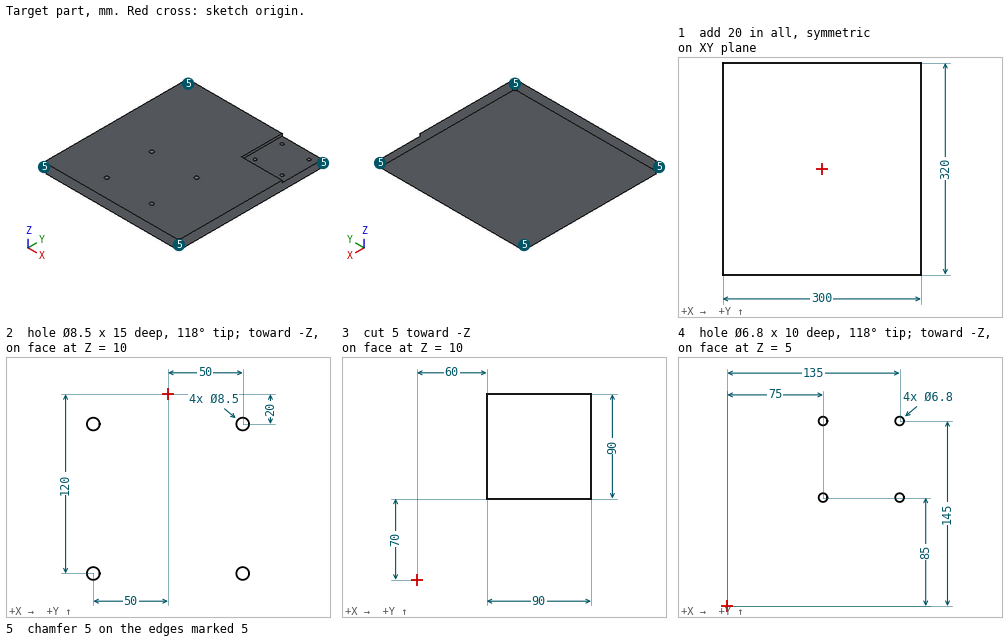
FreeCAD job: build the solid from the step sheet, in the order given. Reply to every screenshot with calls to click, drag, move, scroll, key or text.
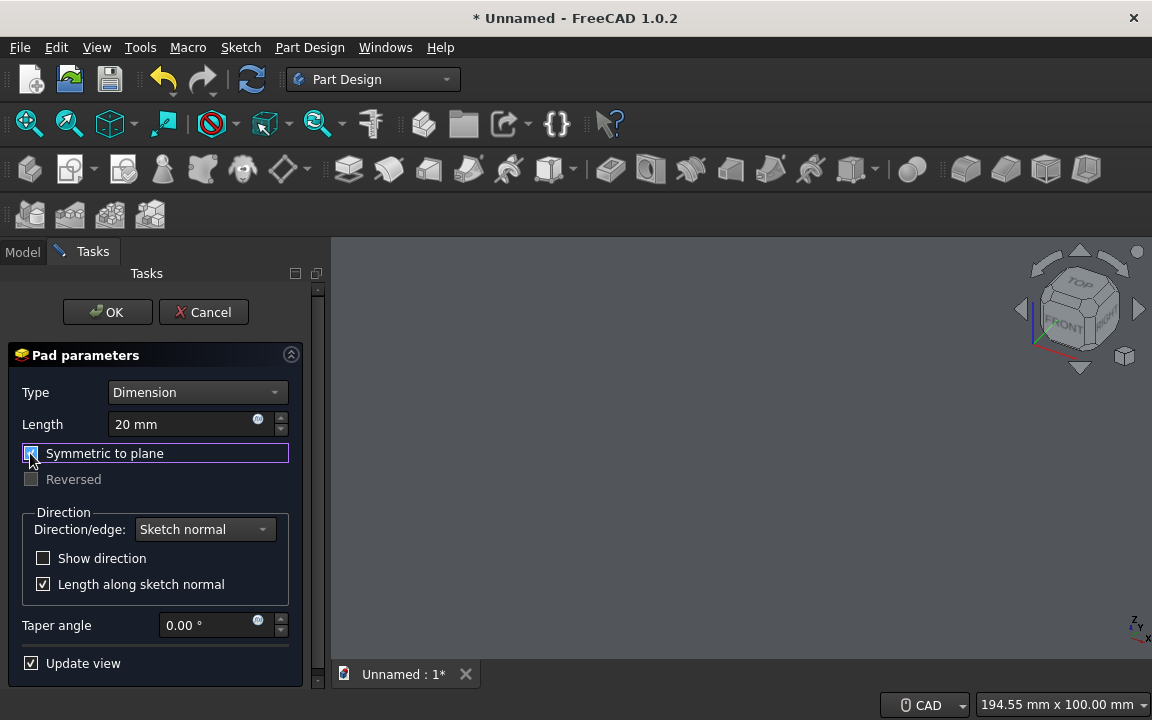
click(108, 312)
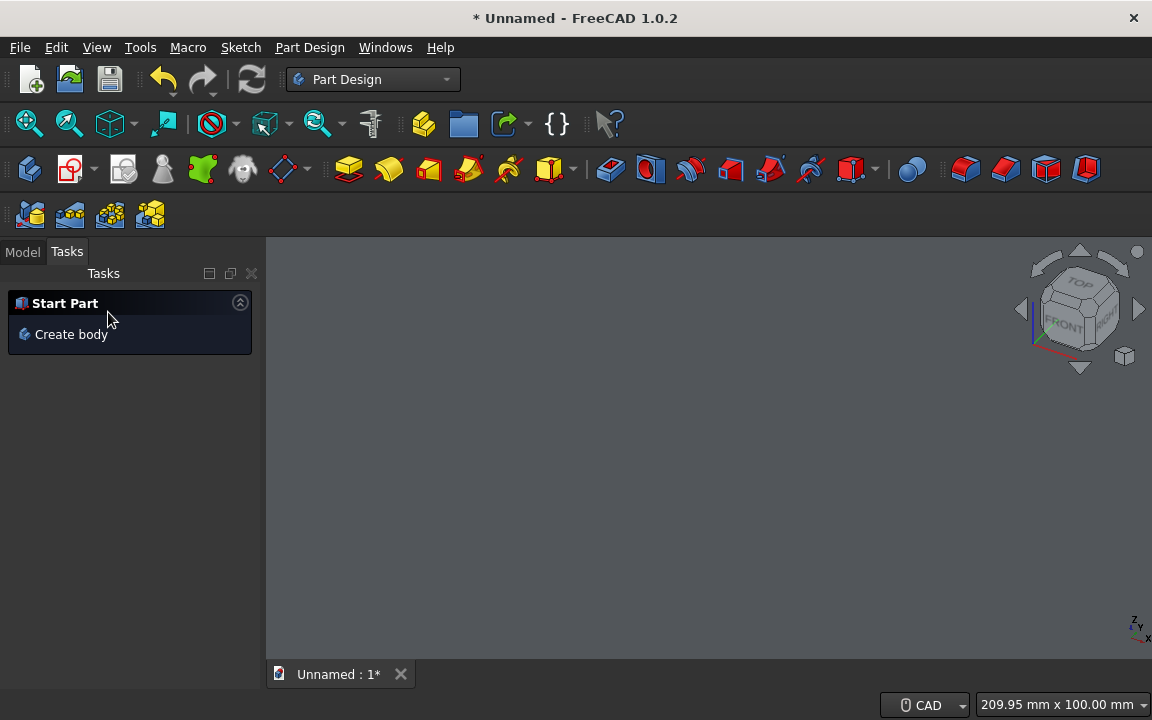
key(v)
key(f)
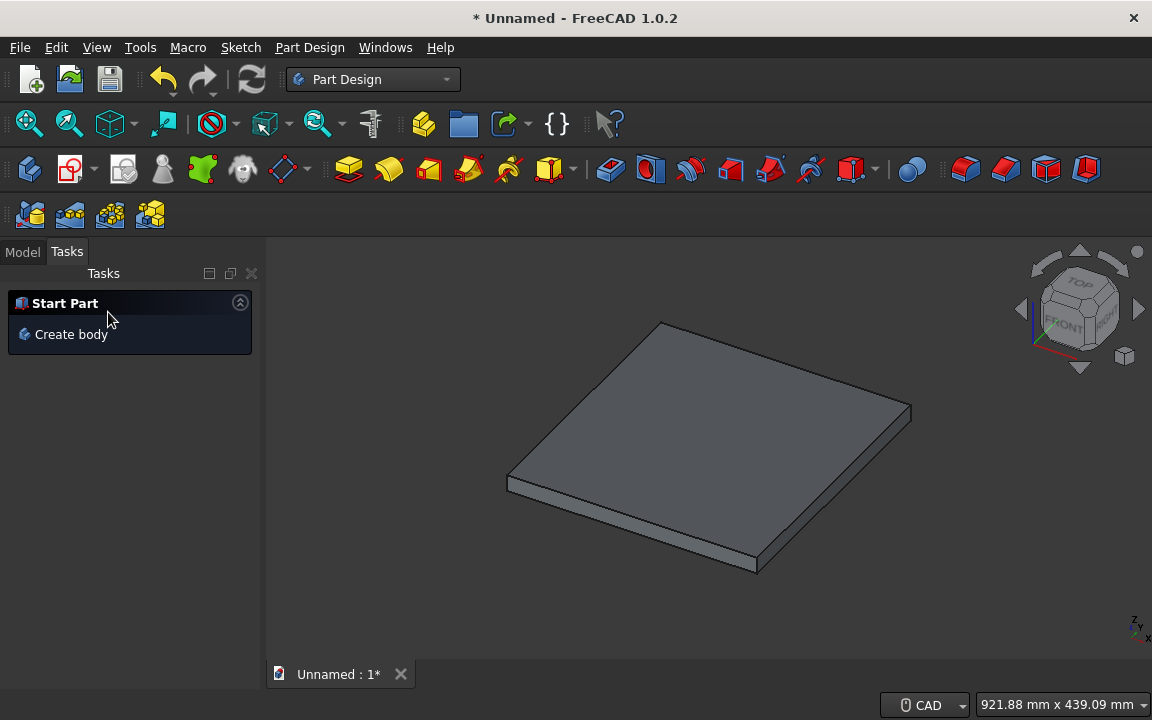
click(709, 439)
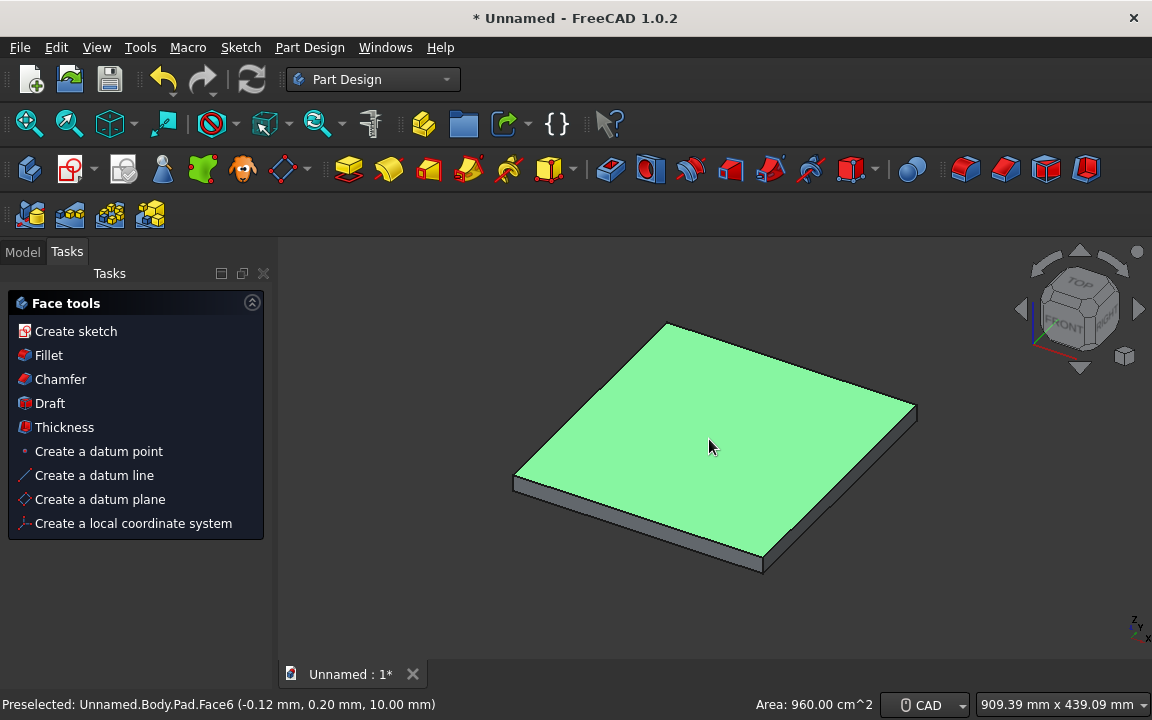
click(70, 170)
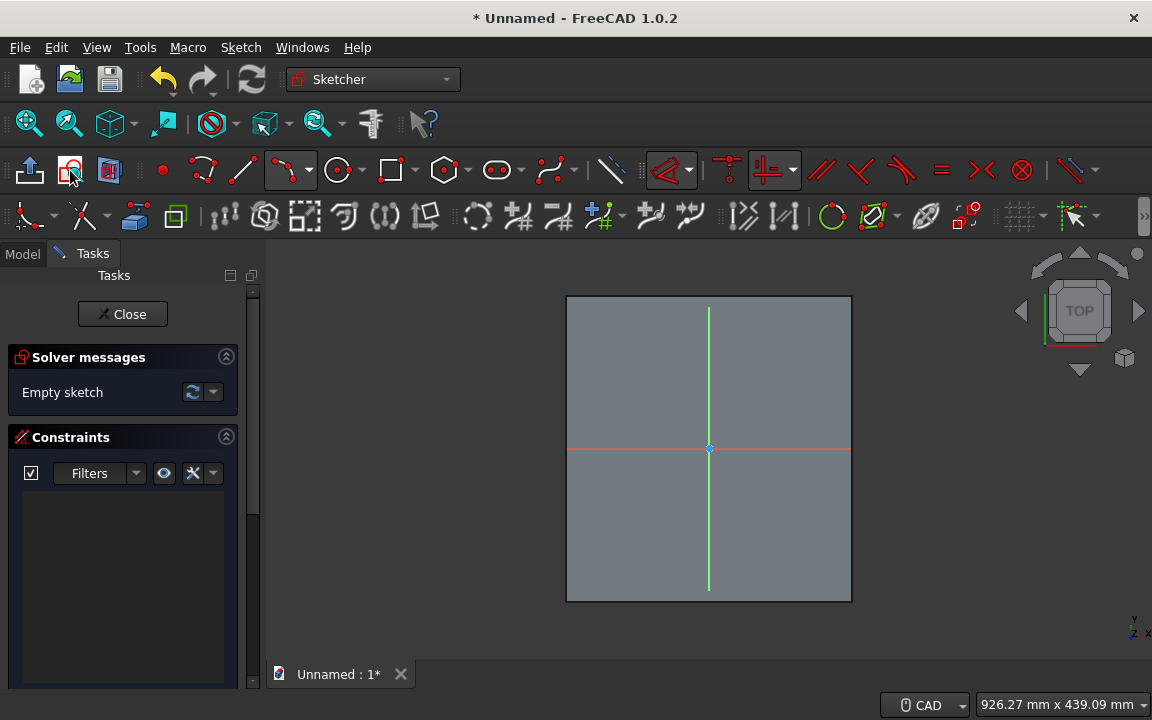
scroll(765, 557, up, 4)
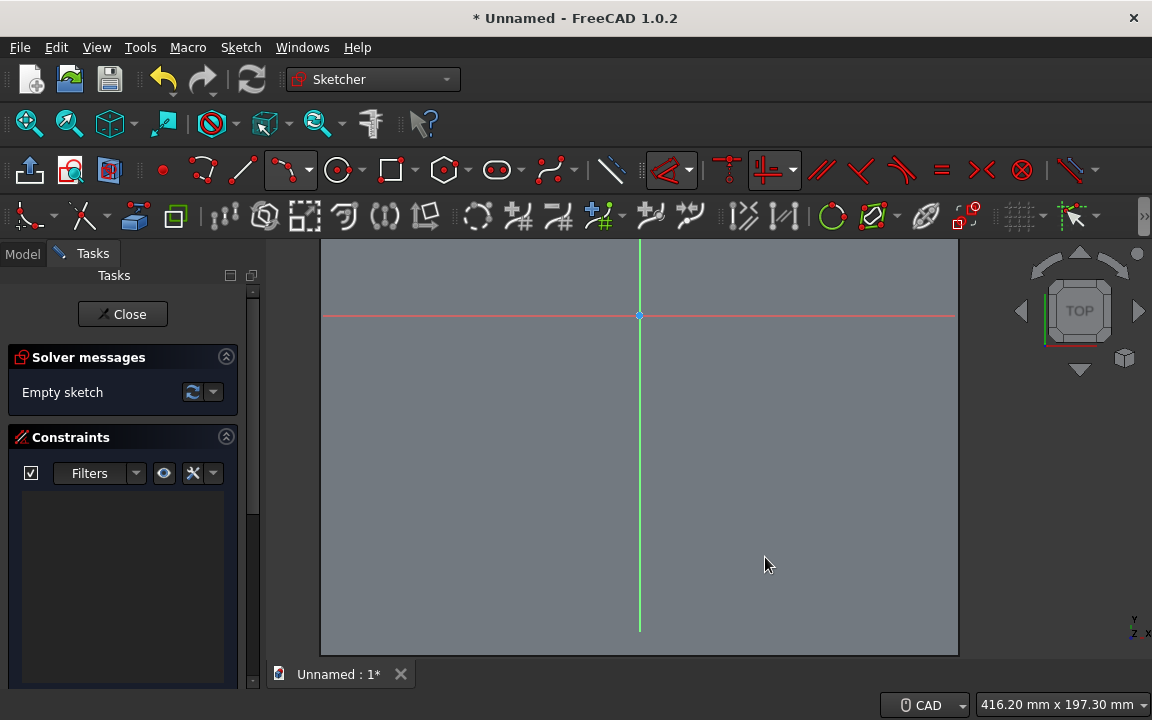
key(g)
key(c)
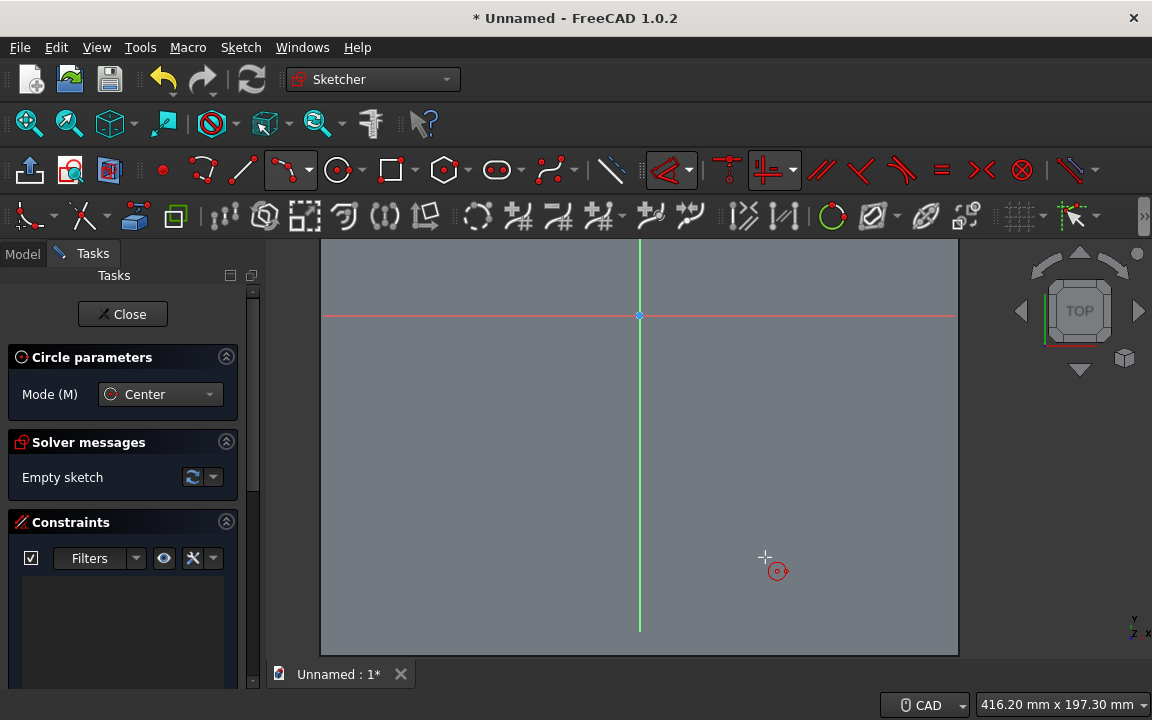
scroll(746, 358, up, 5)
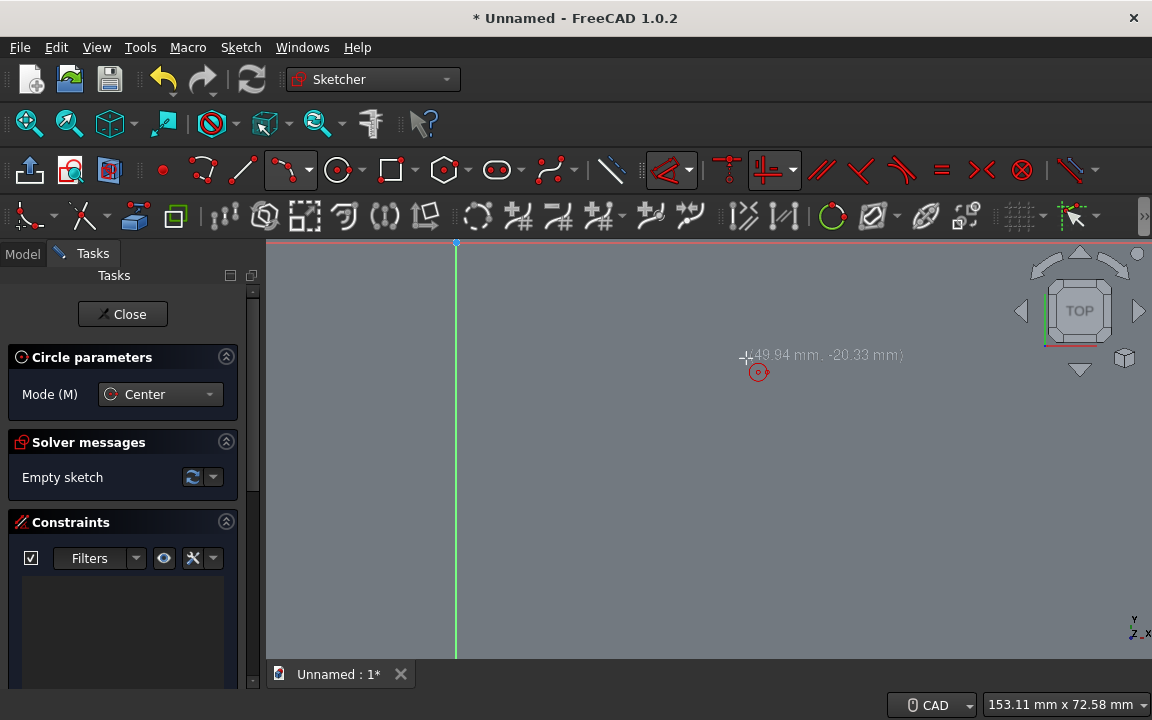
click(745, 358)
move(763, 341)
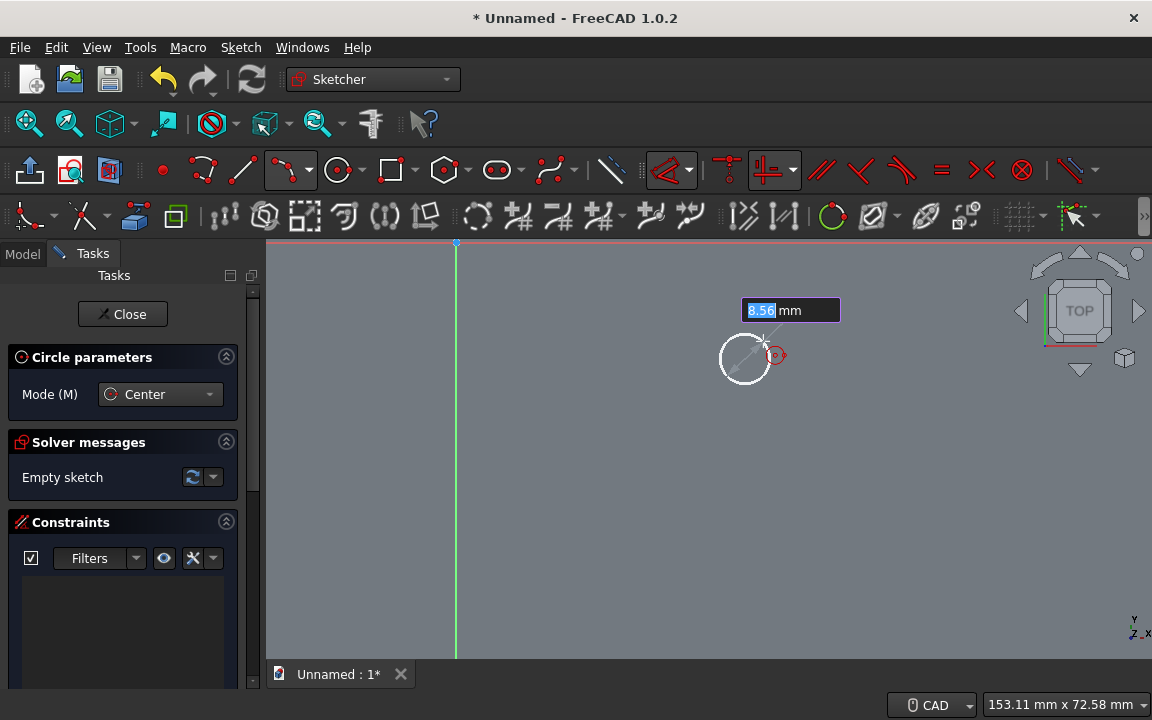
text(8.5)
key(Return)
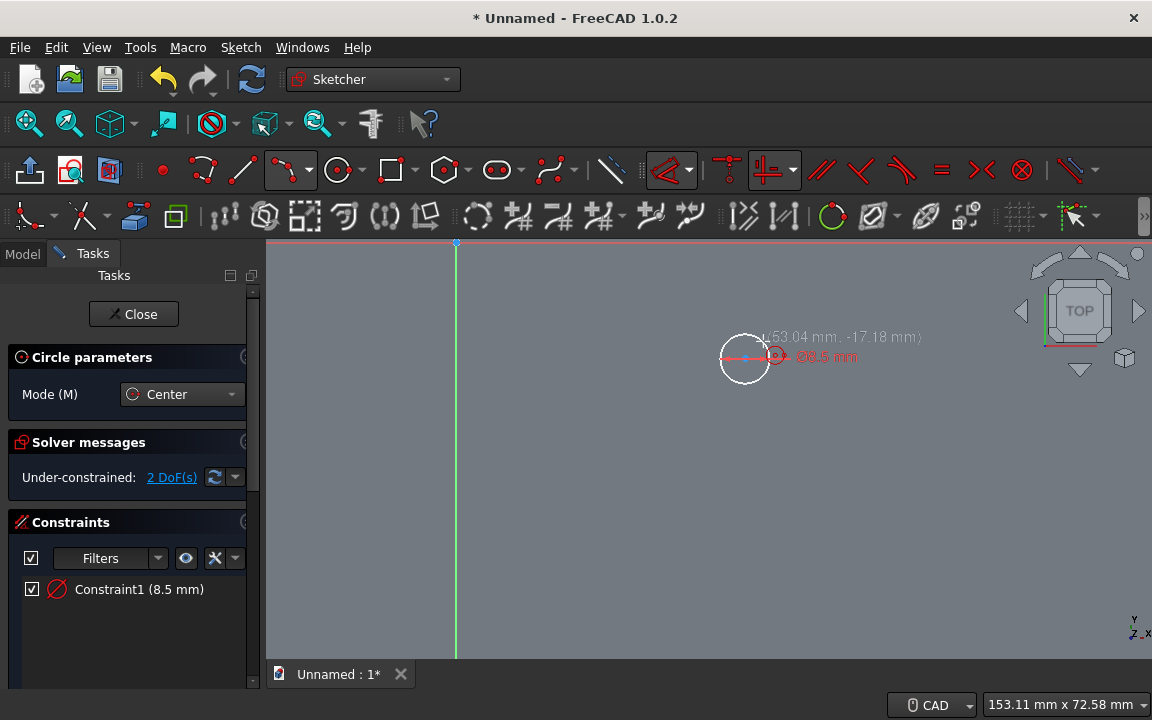
scroll(748, 360, down, 5)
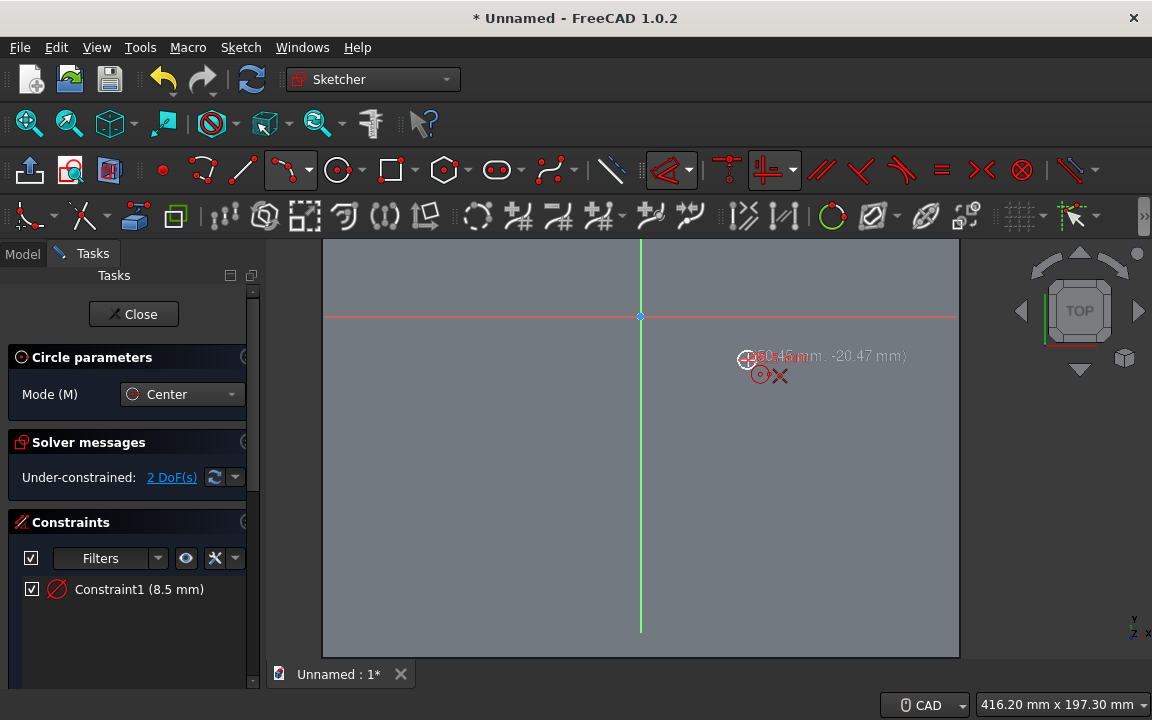
scroll(535, 572, up, 5)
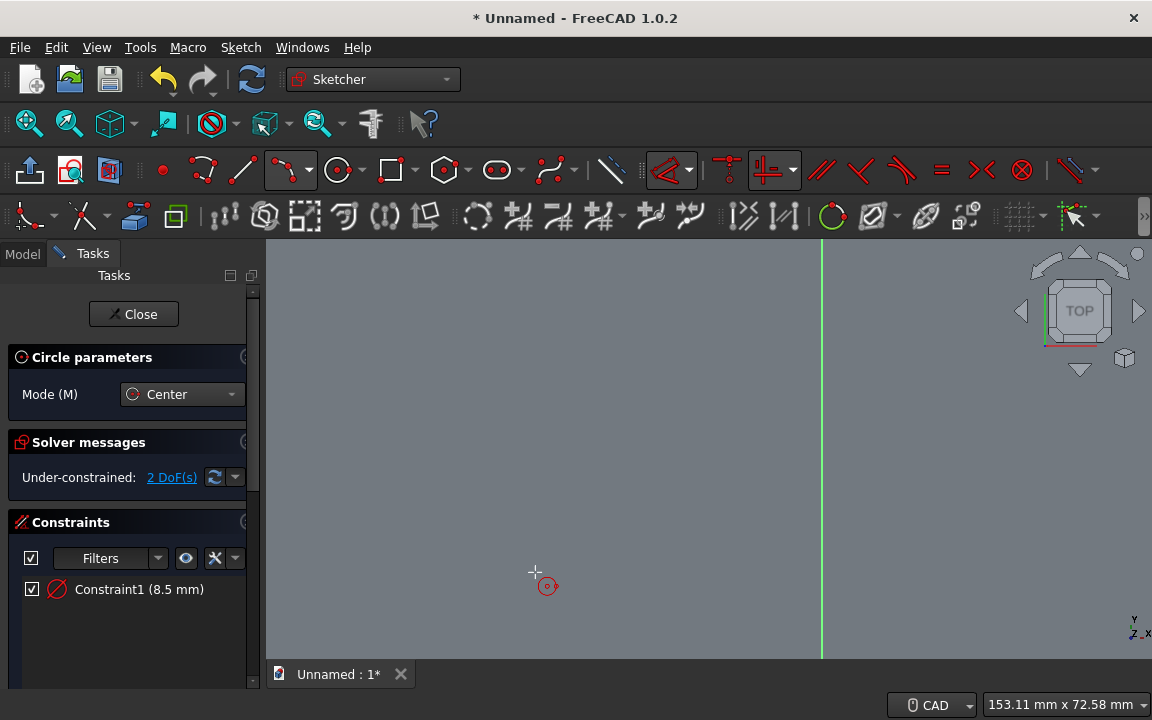
click(533, 572)
move(551, 554)